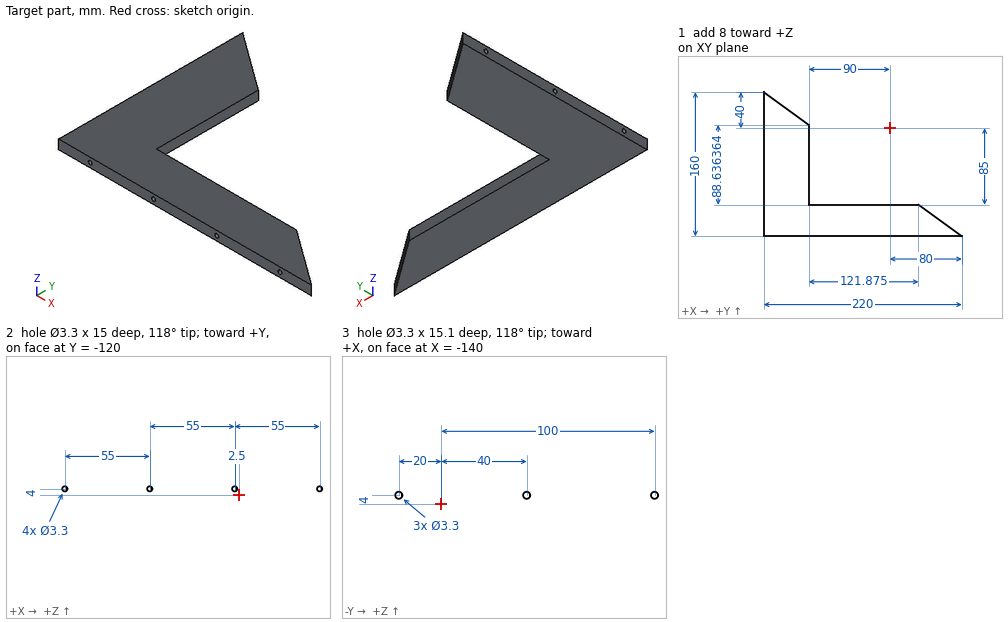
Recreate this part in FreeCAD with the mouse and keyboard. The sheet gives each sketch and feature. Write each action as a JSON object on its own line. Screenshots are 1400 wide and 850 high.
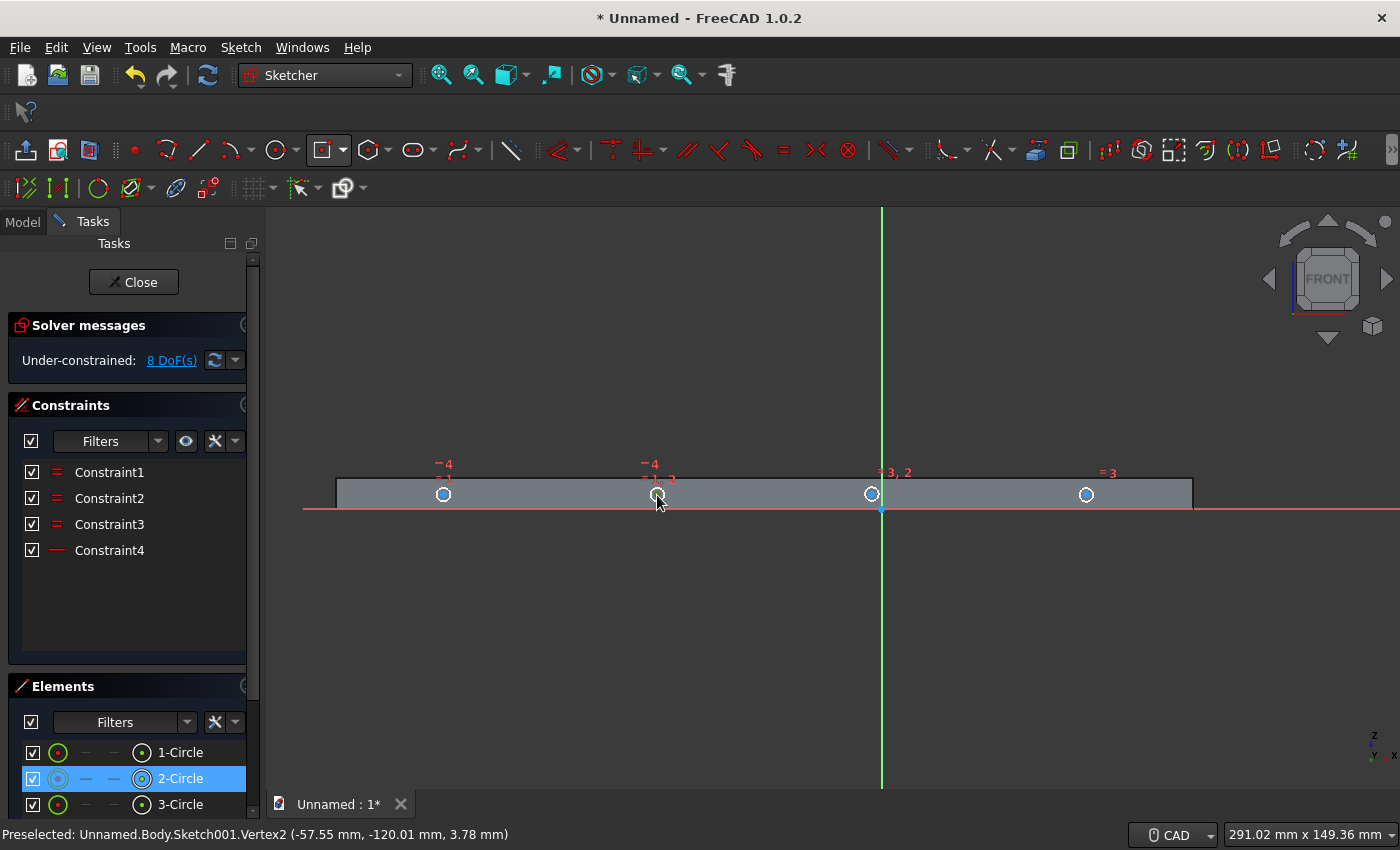
{"action": "left_click", "coordinate": [872, 494]}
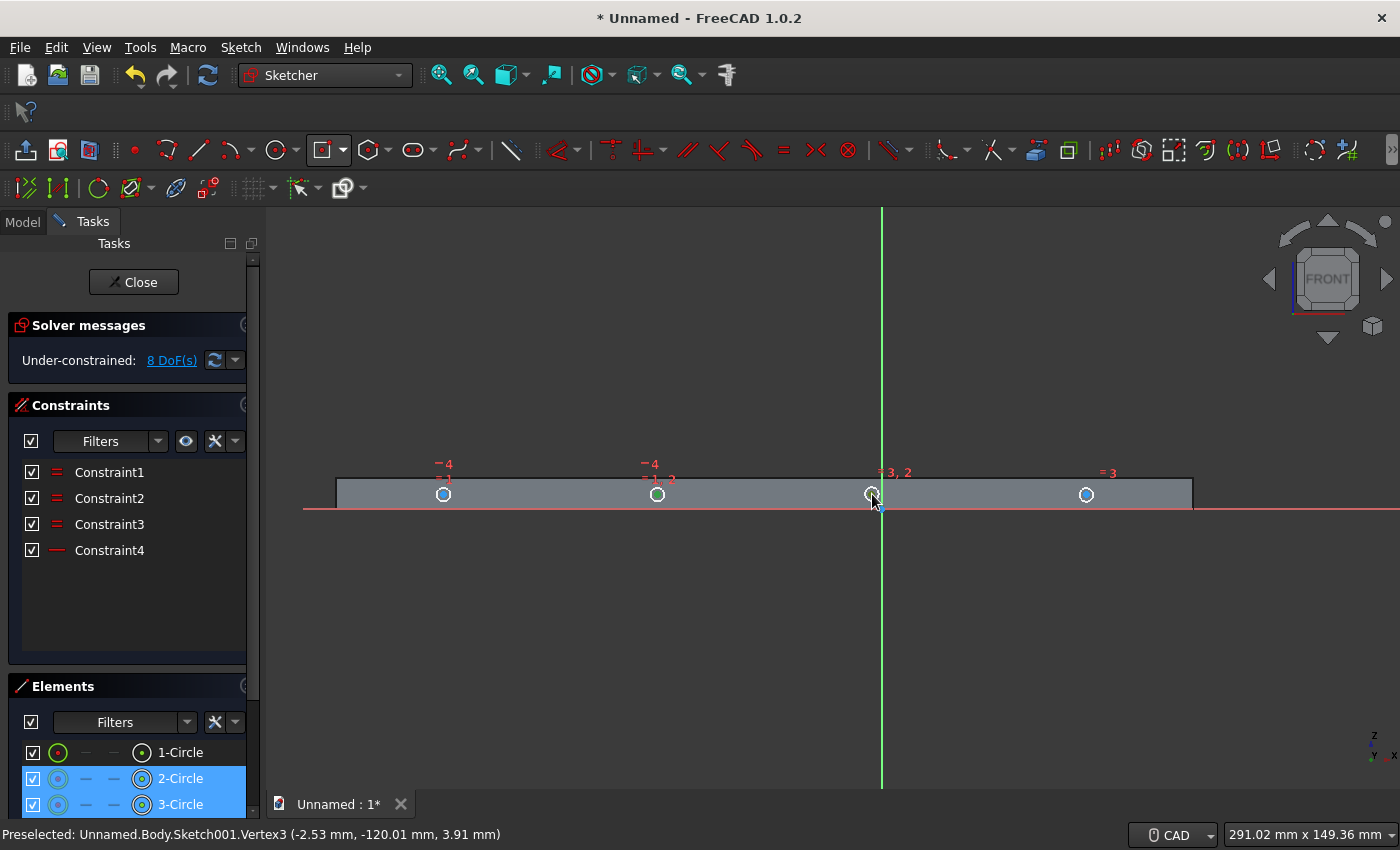
{"action": "key", "text": "h"}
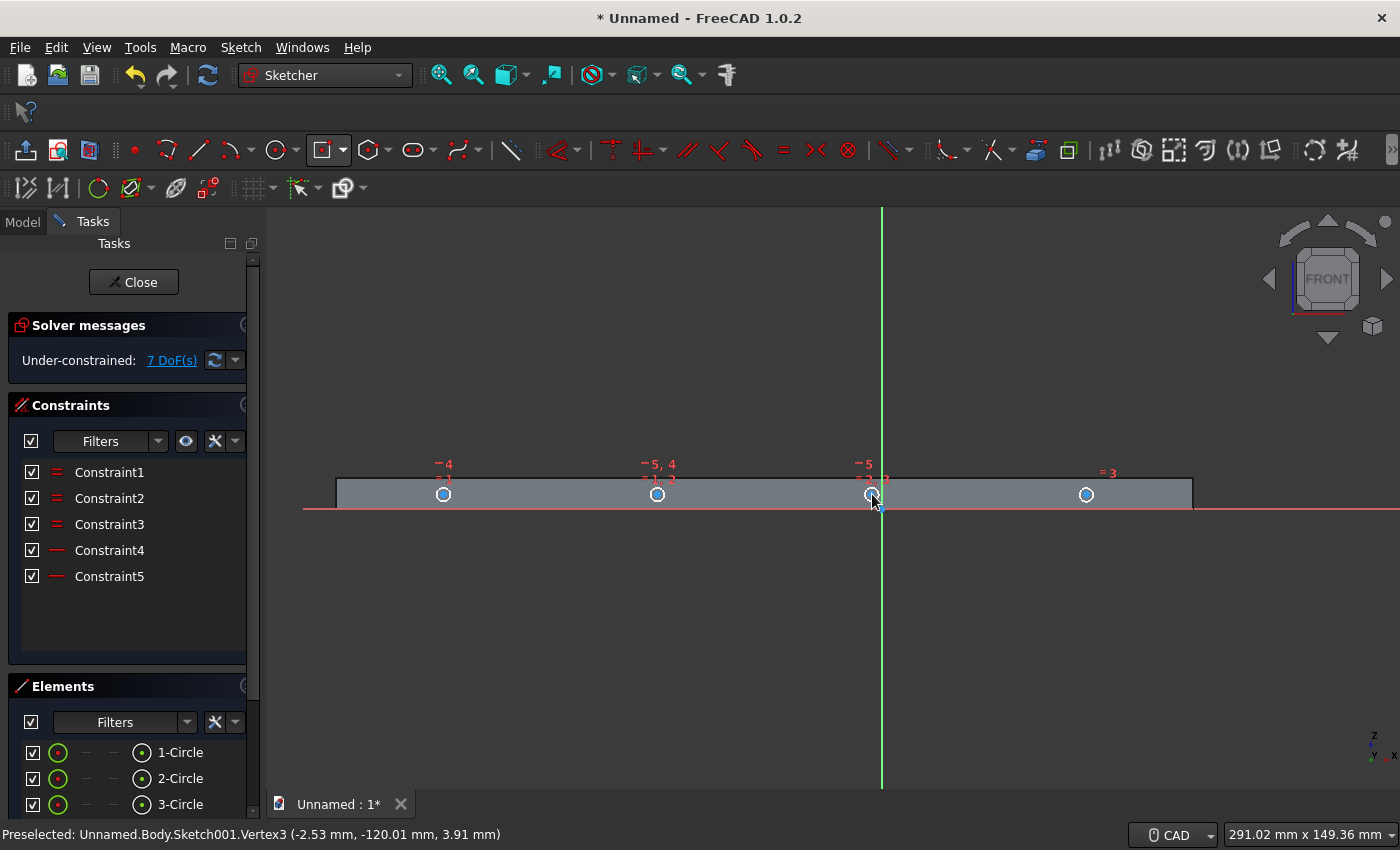
{"action": "left_click", "coordinate": [872, 495]}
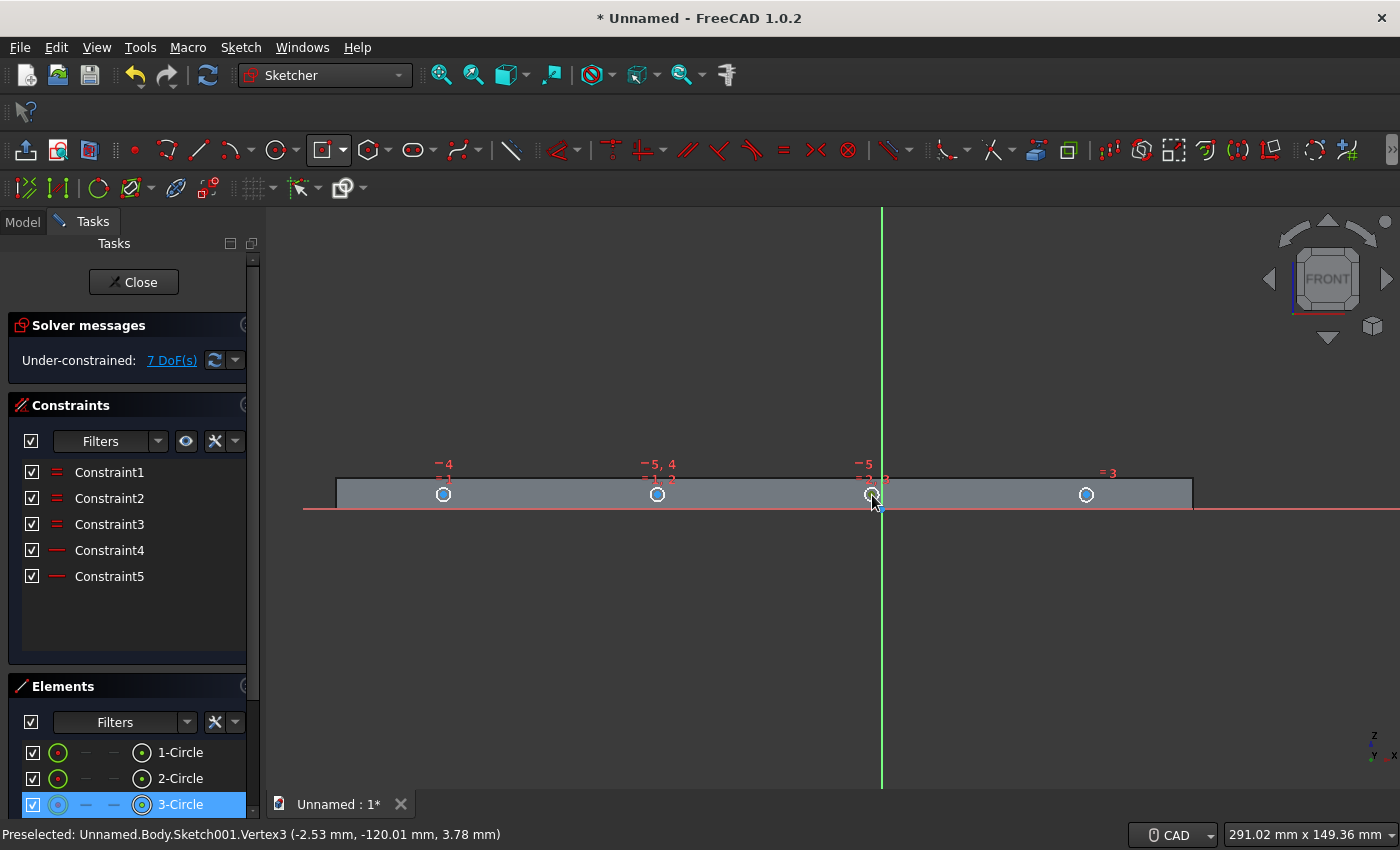
{"action": "left_click", "coordinate": [1086, 495]}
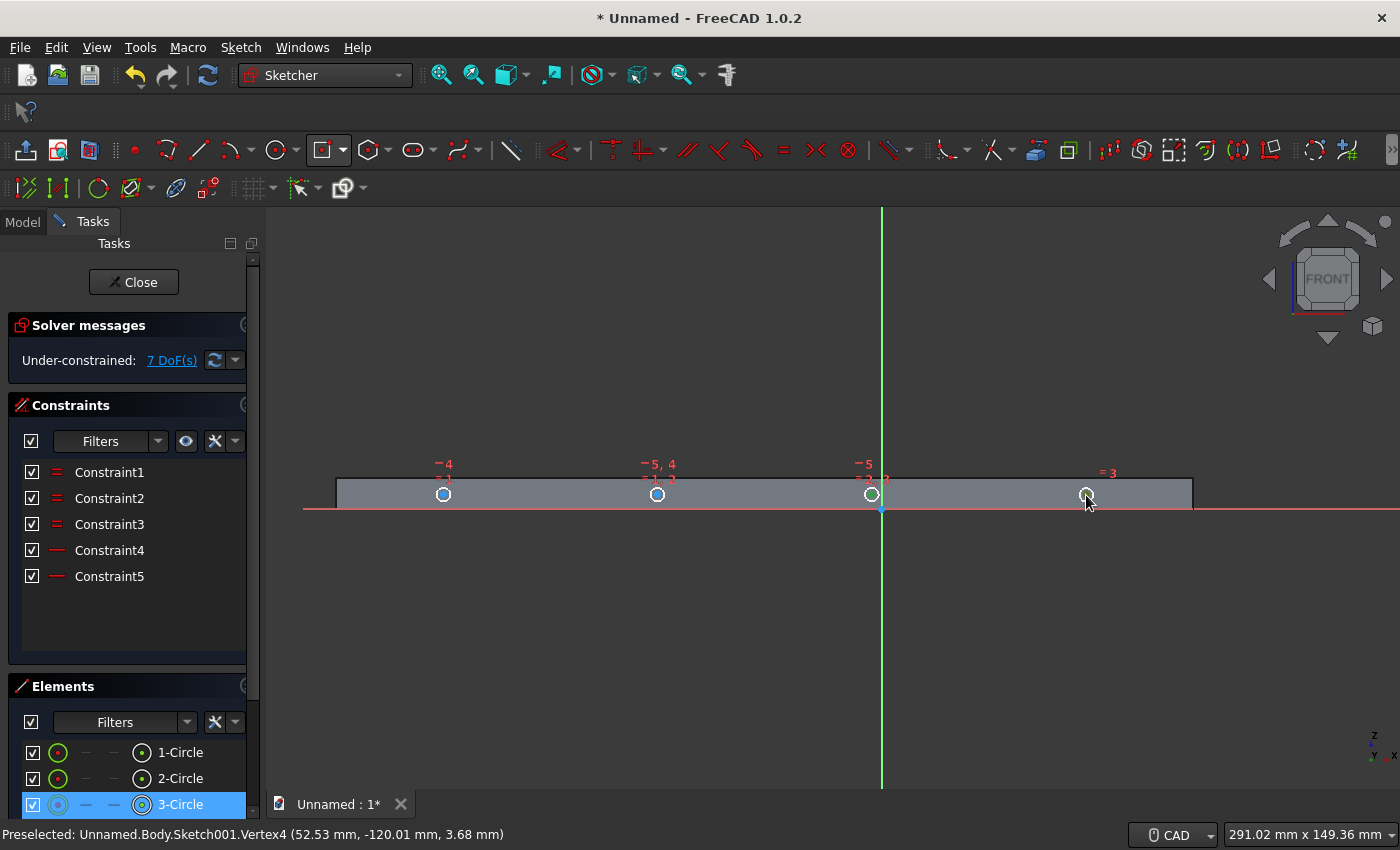
{"action": "key", "text": "h"}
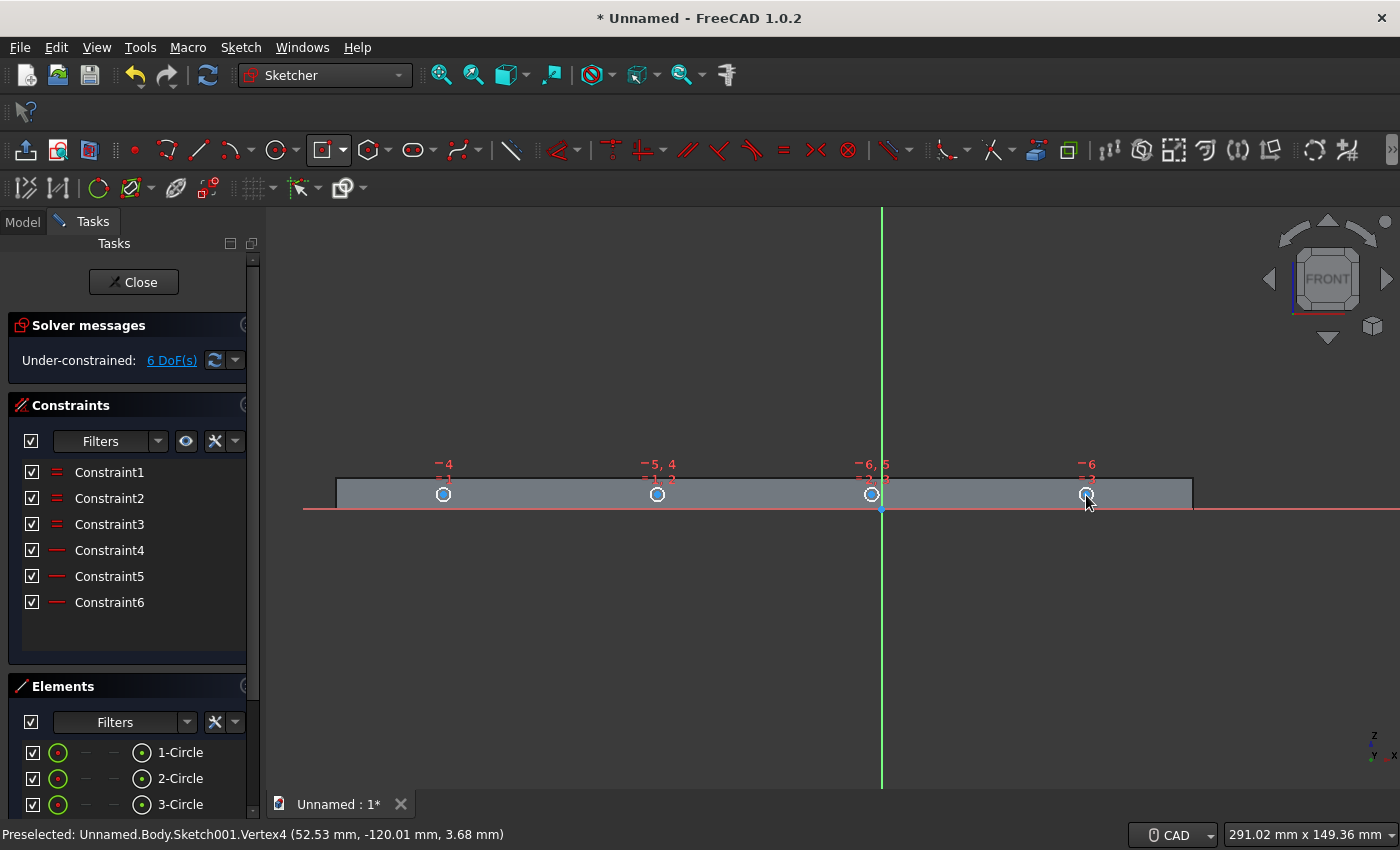
{"action": "key", "text": "d"}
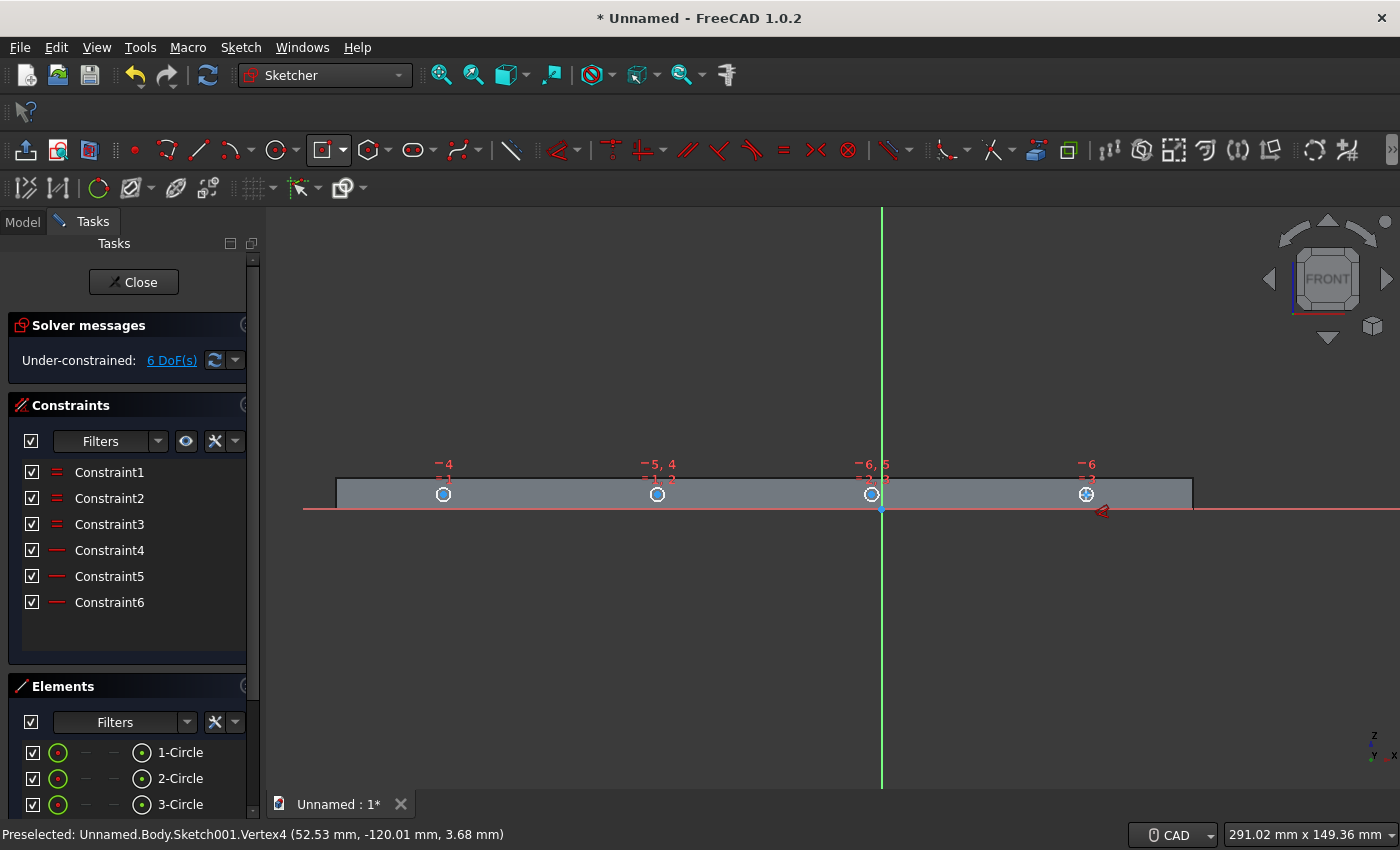
{"action": "scroll", "coordinate": [448, 499], "scroll_direction": "up", "scroll_amount": 6}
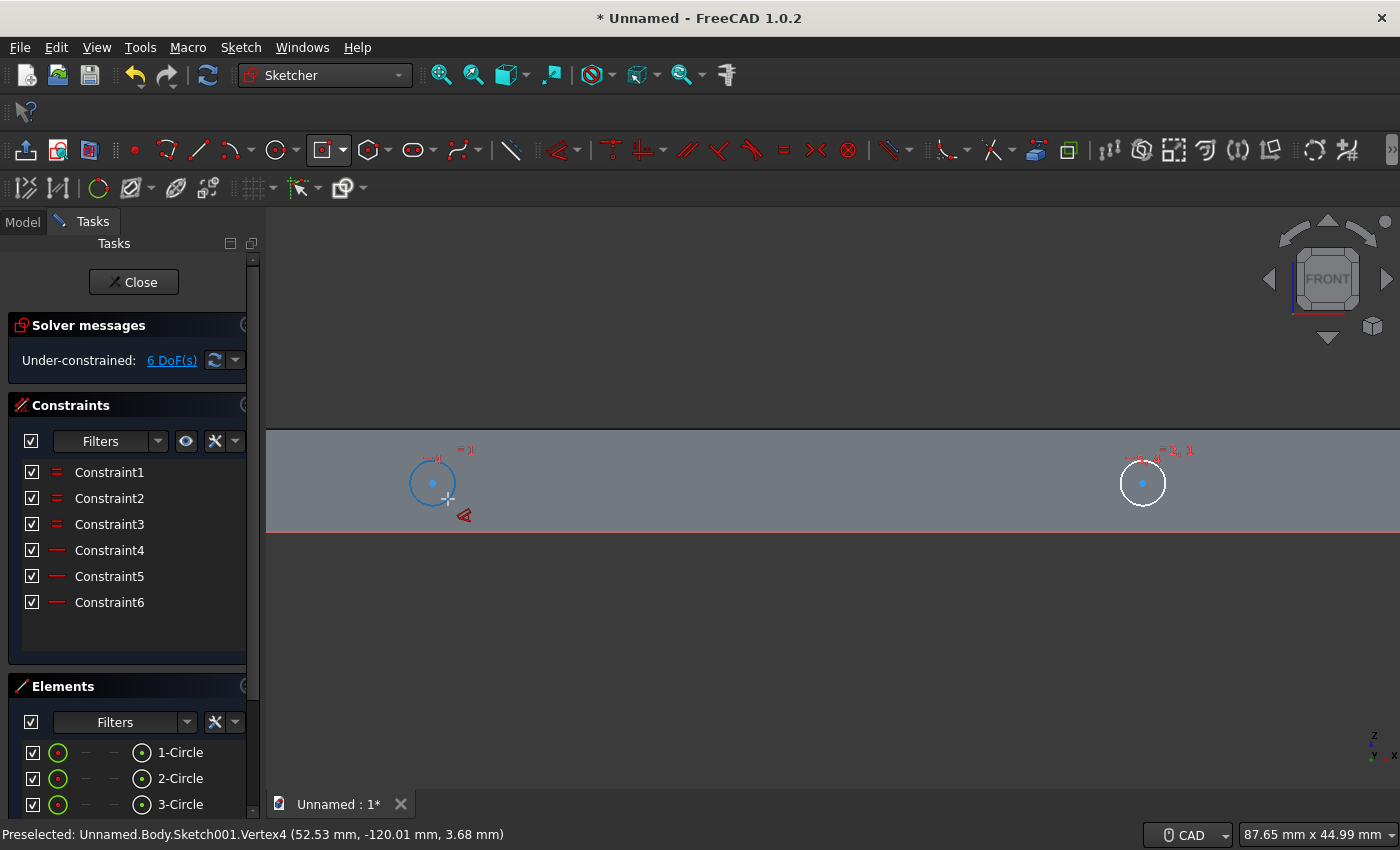
{"action": "left_click", "coordinate": [449, 499]}
{"action": "left_click", "coordinate": [485, 498]}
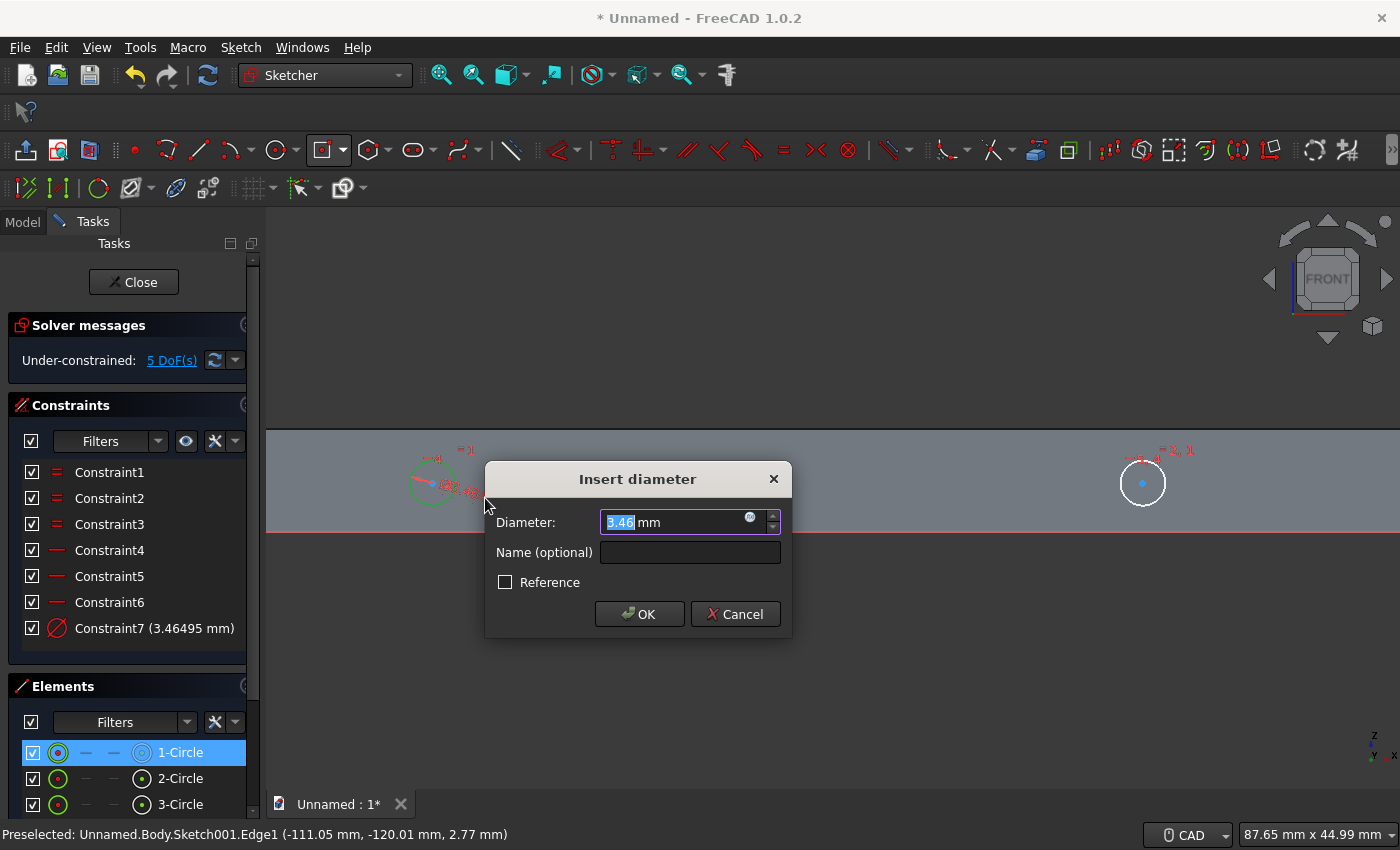
{"action": "type", "text": "3.3"}
{"action": "key", "text": "Return"}